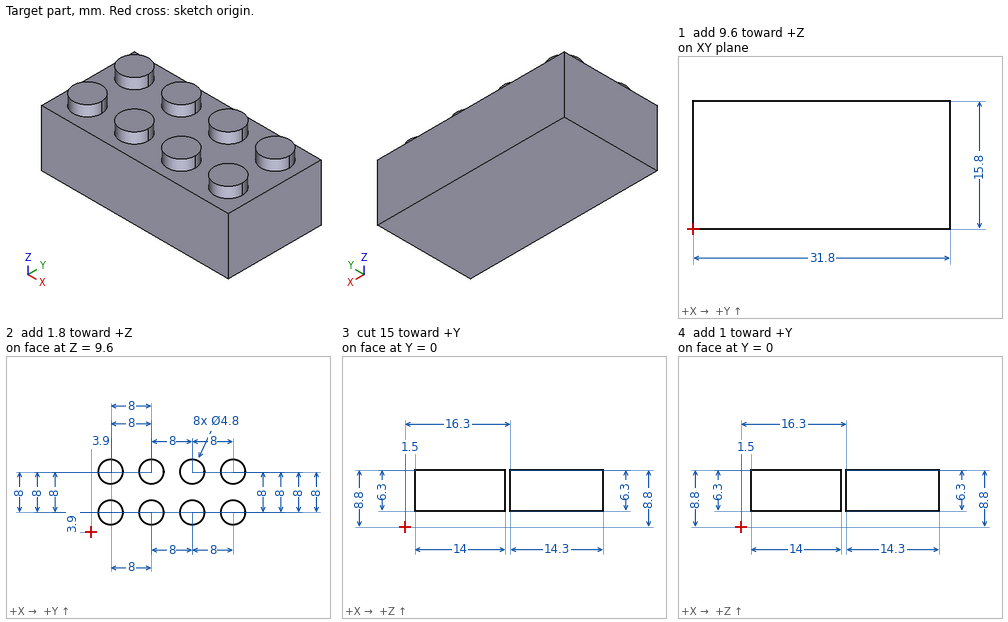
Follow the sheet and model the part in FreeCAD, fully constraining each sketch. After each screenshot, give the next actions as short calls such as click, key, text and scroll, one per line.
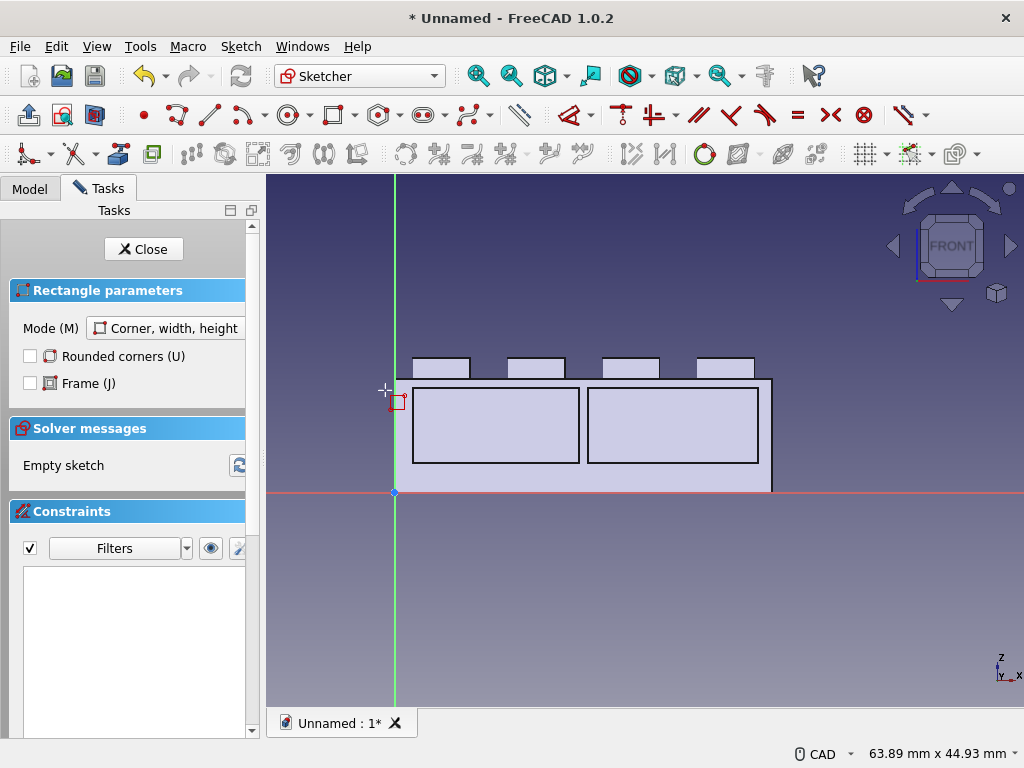
click(413, 388)
click(579, 463)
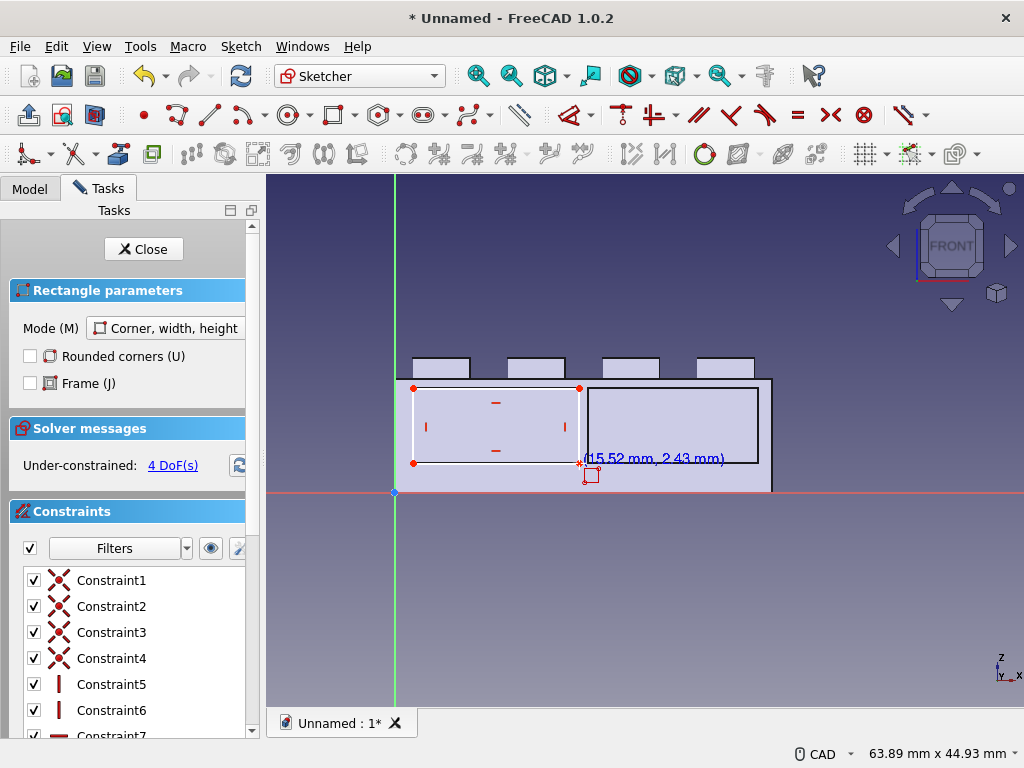
scroll(588, 388, up, 3)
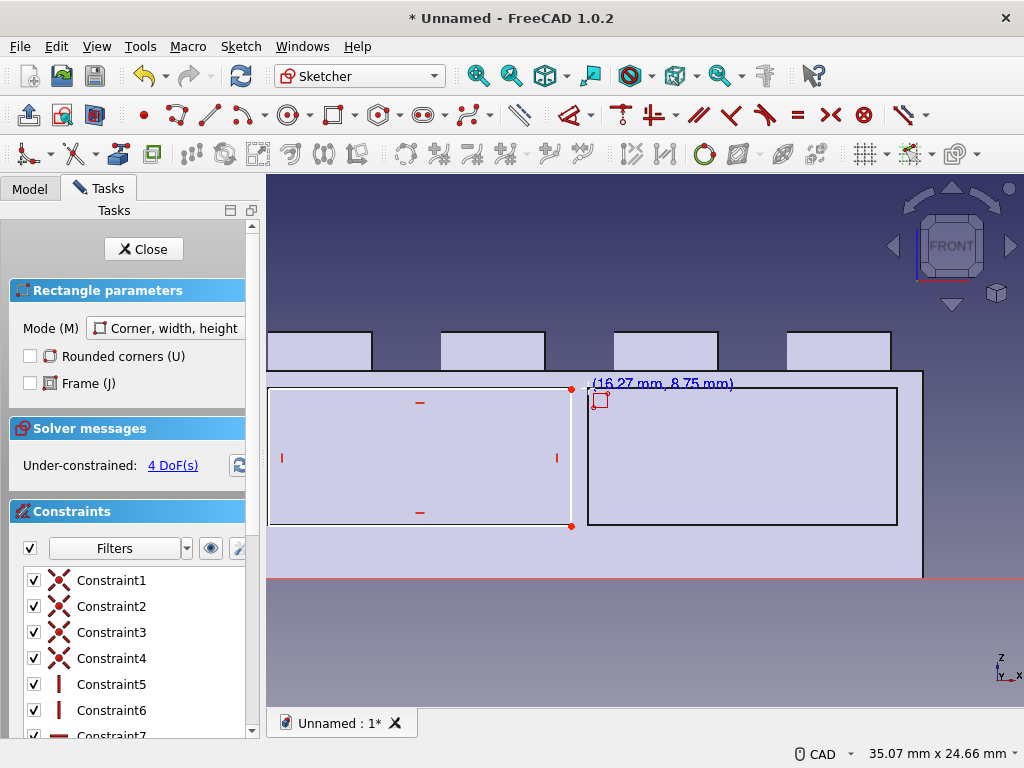
click(588, 388)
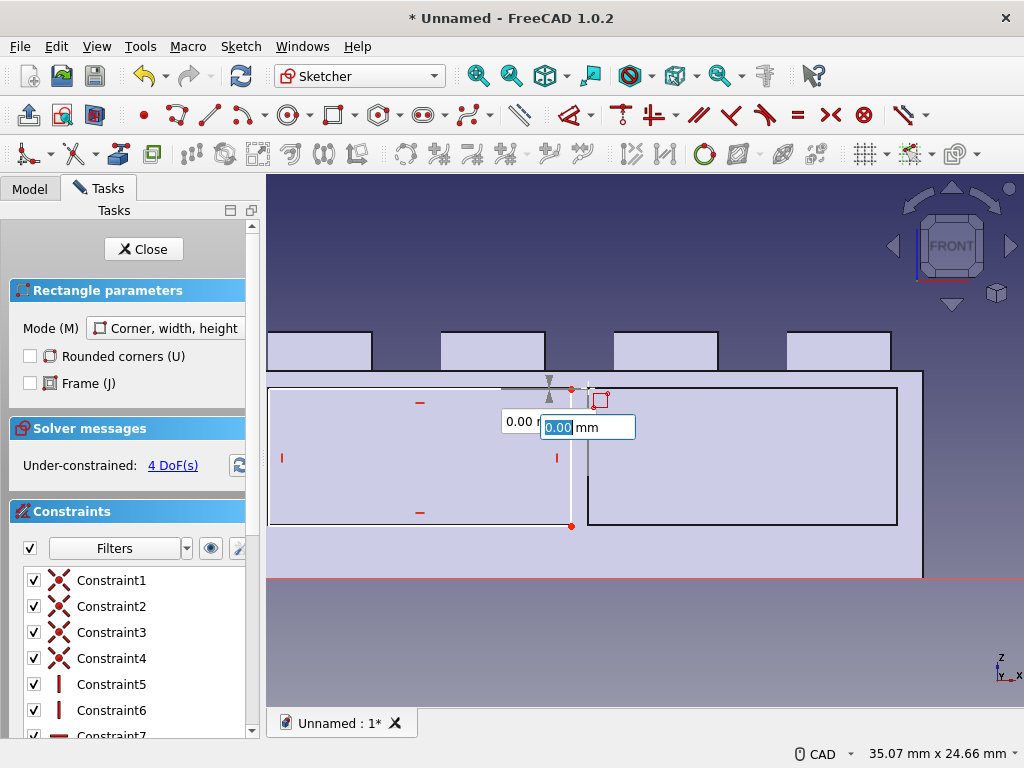
scroll(589, 388, down, 3)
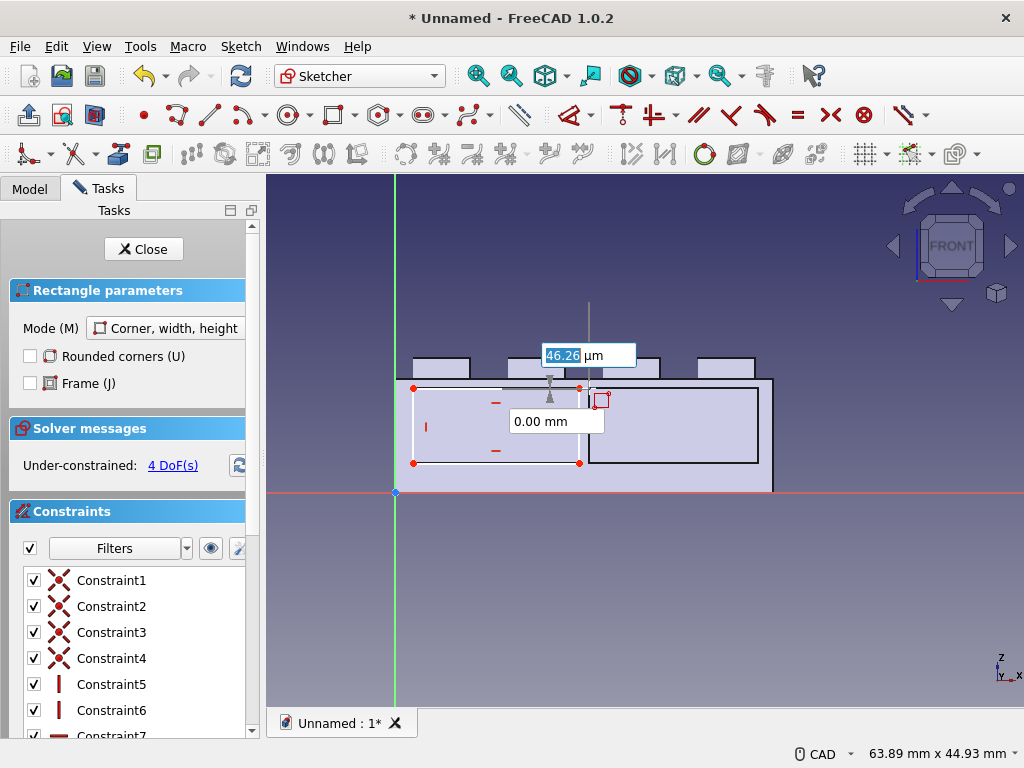
click(758, 463)
key(Escape)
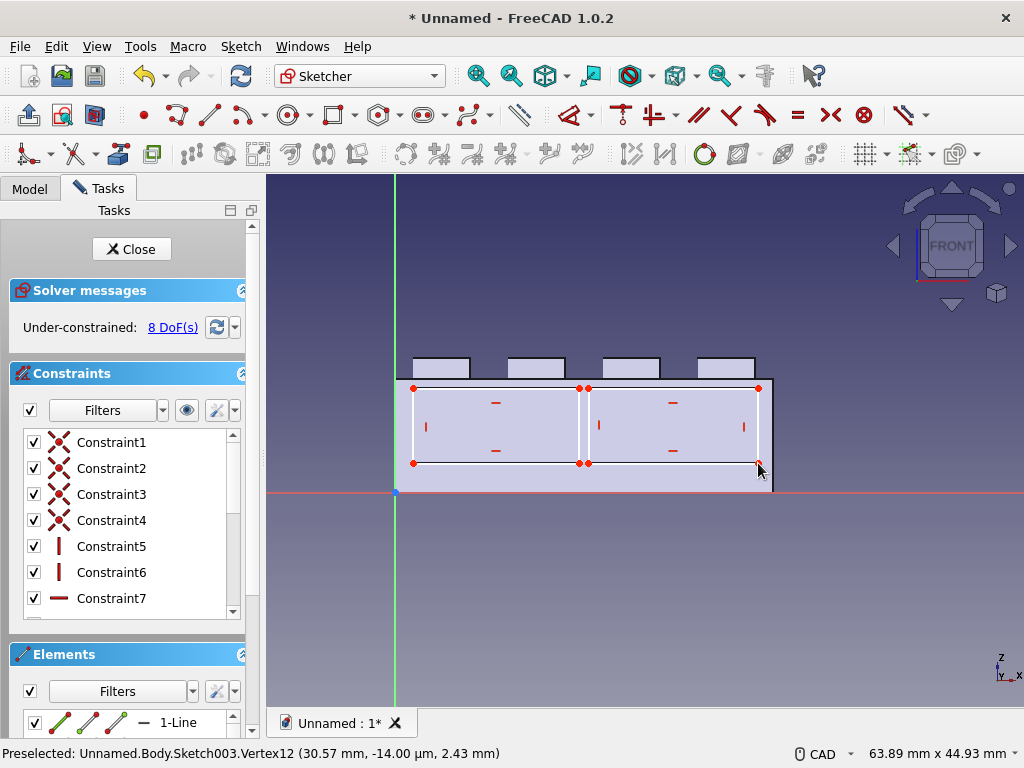
key(d)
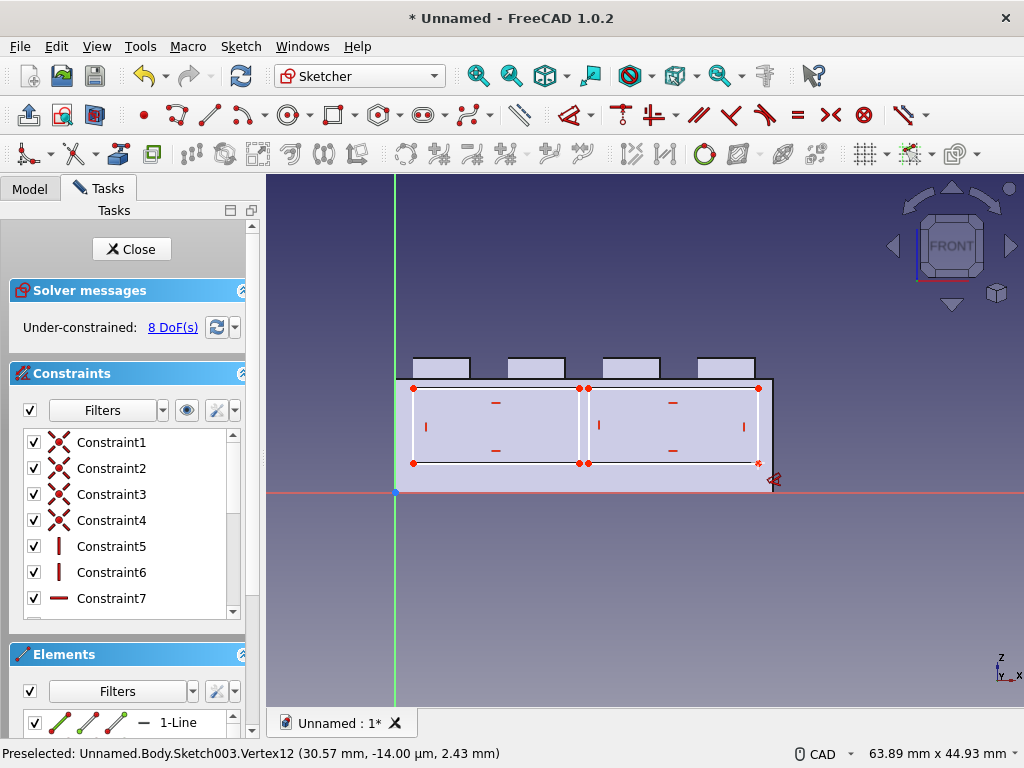
click(463, 464)
click(496, 430)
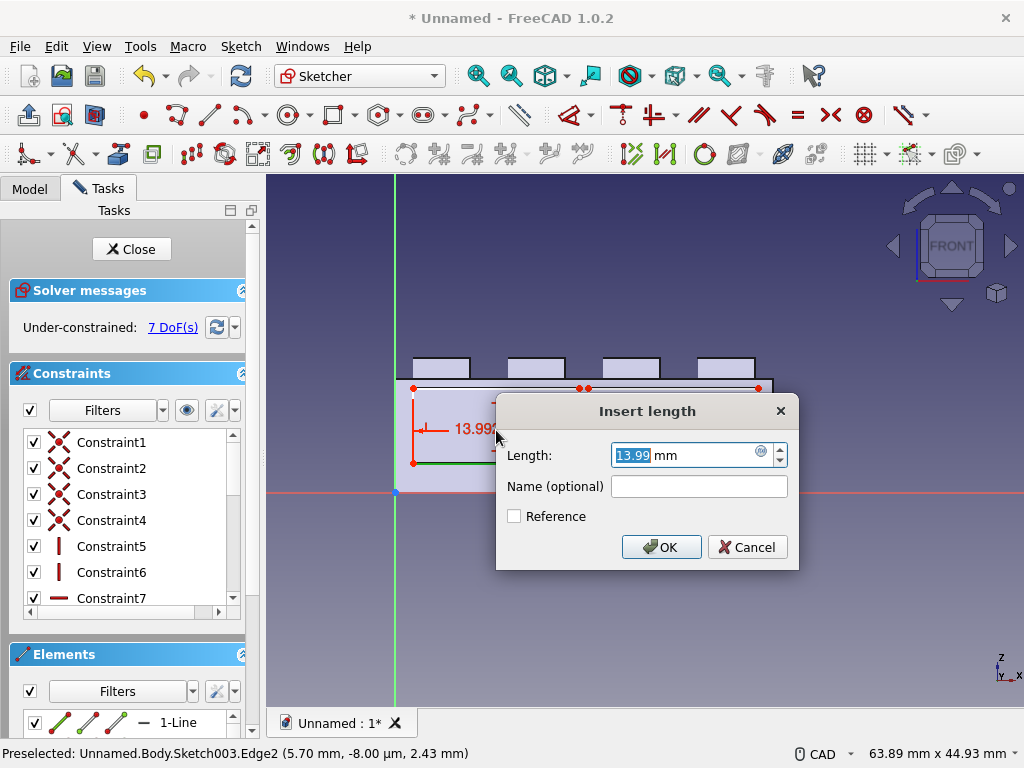
text(14)
key(Return)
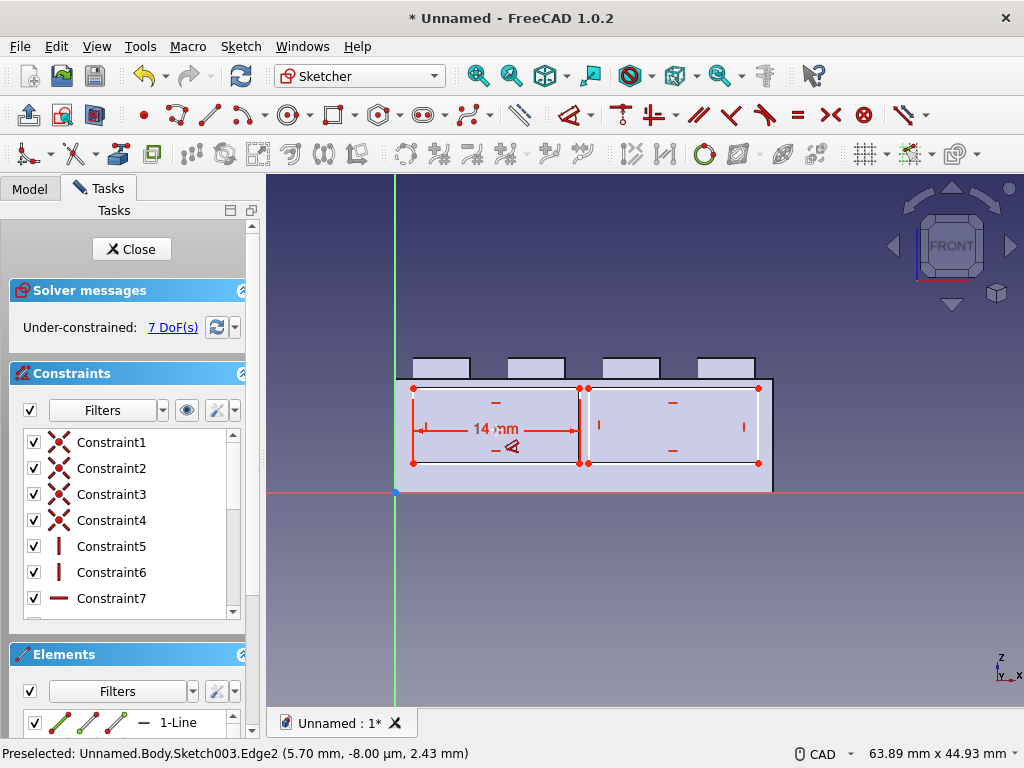
click(413, 411)
click(379, 426)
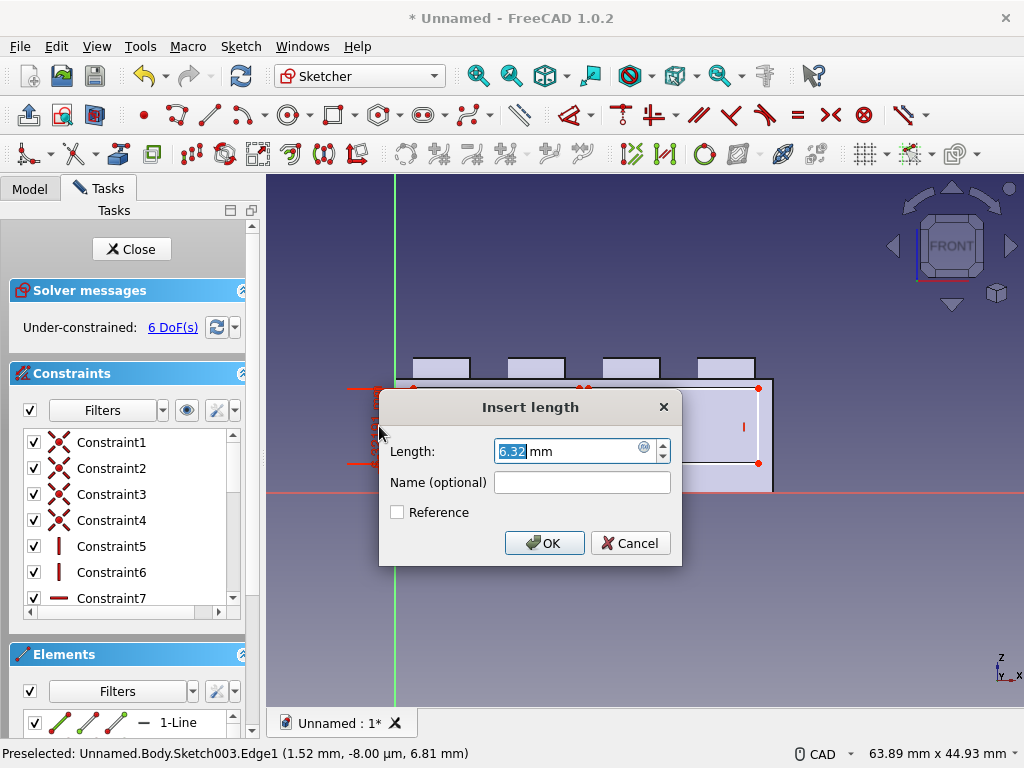
text(6.3)
key(Return)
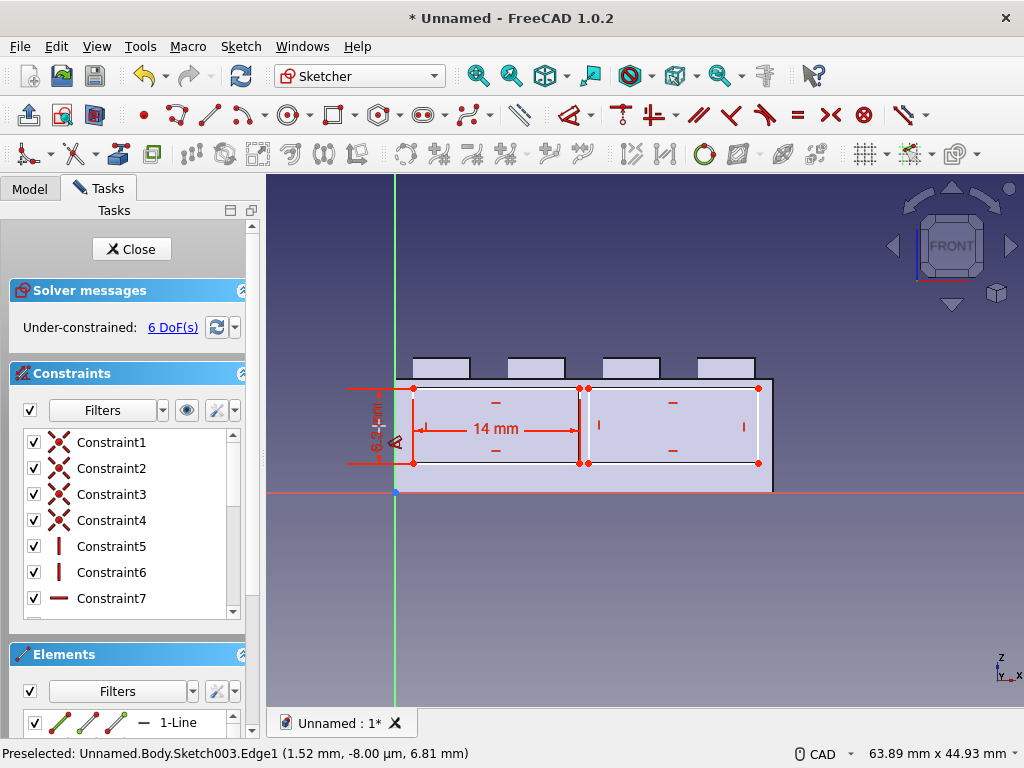
scroll(589, 411, up, 3)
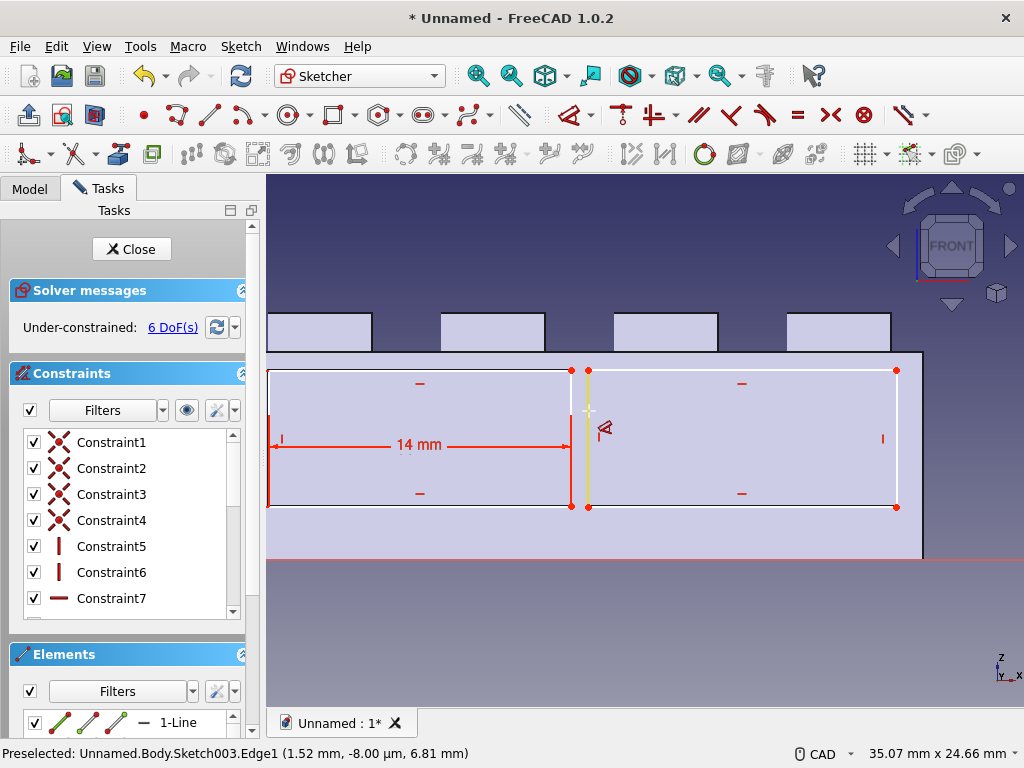
click(588, 411)
click(622, 439)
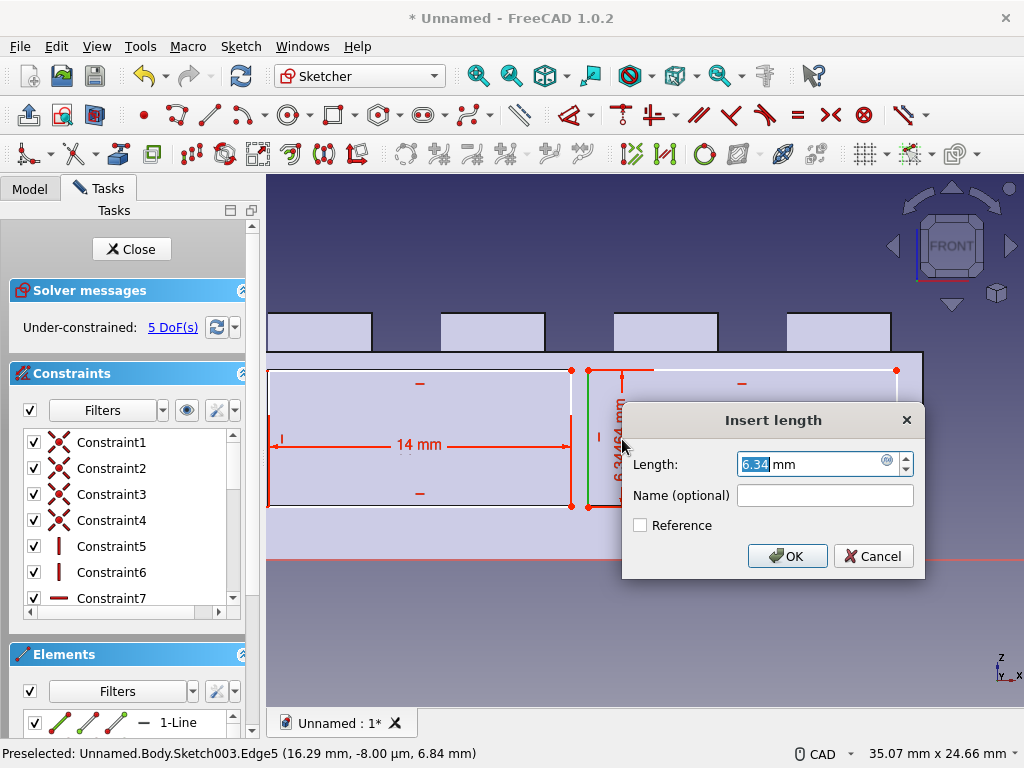
text(6.3)
key(Return)